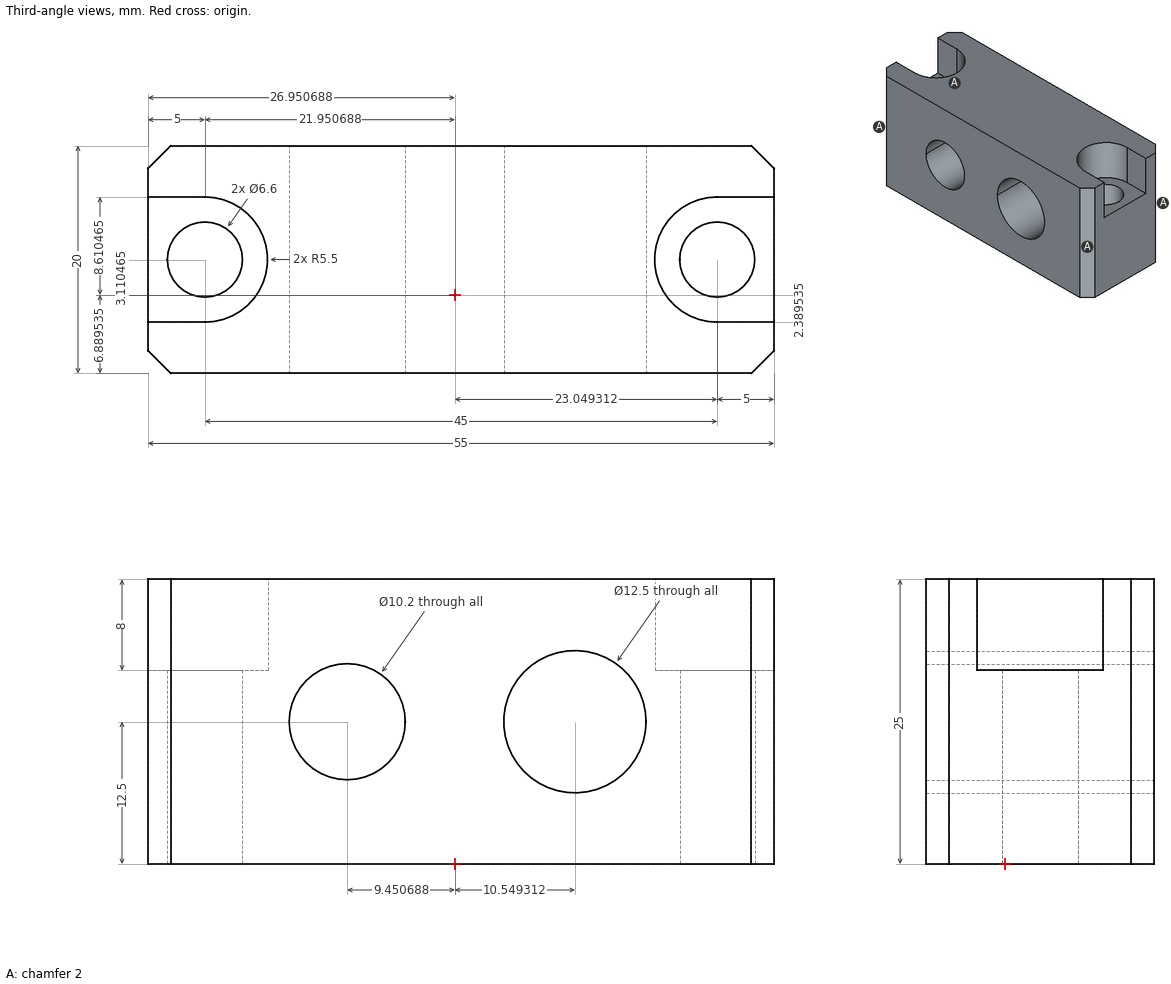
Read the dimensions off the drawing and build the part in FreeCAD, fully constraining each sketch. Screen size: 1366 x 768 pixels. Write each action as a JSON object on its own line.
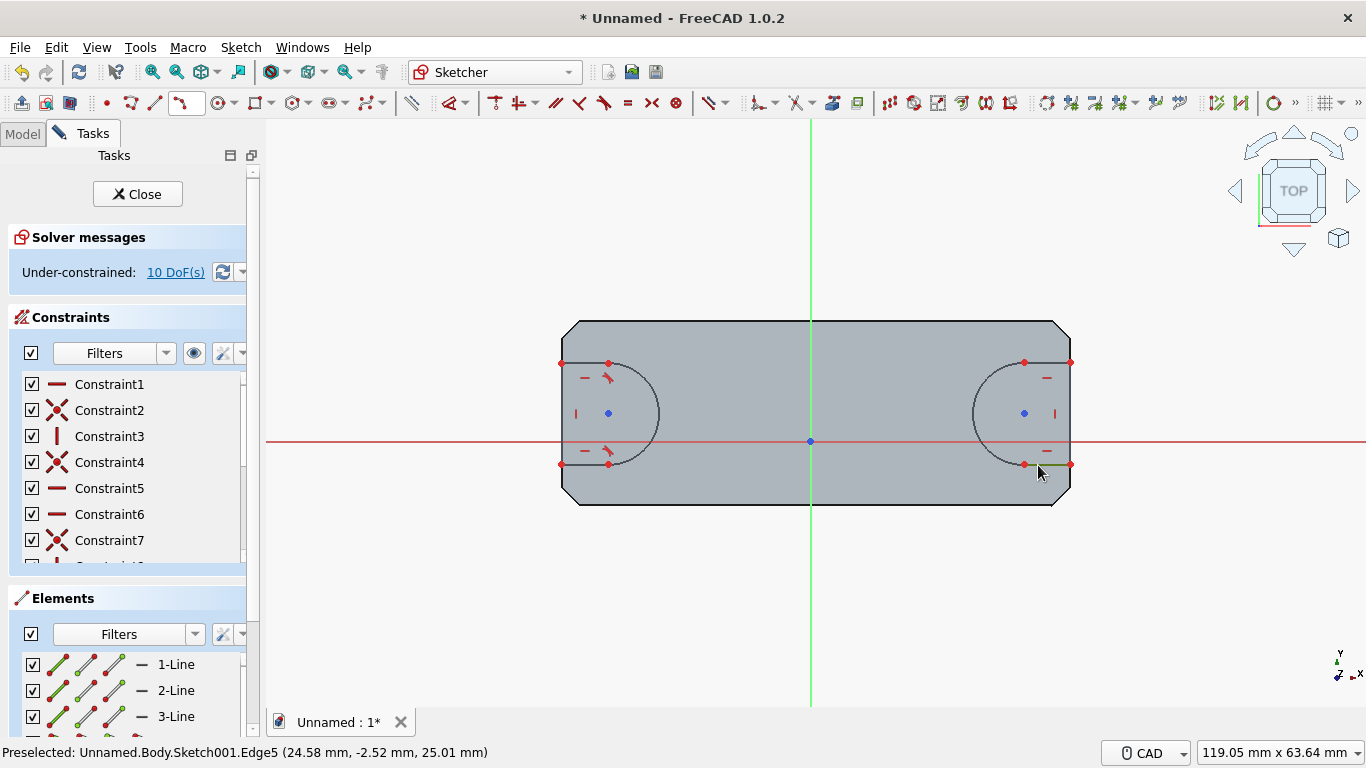
{"action": "left_click", "coordinate": [983, 384]}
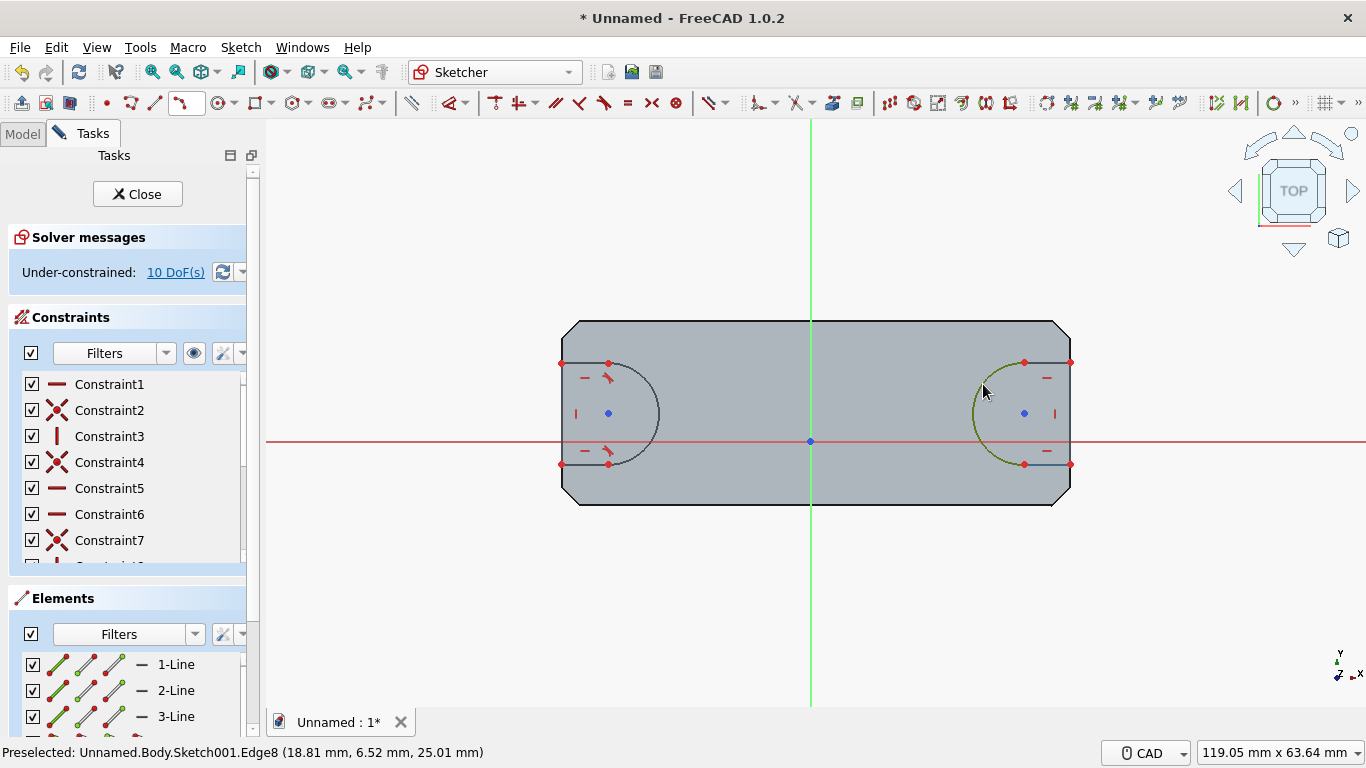
{"action": "left_click", "coordinate": [604, 104]}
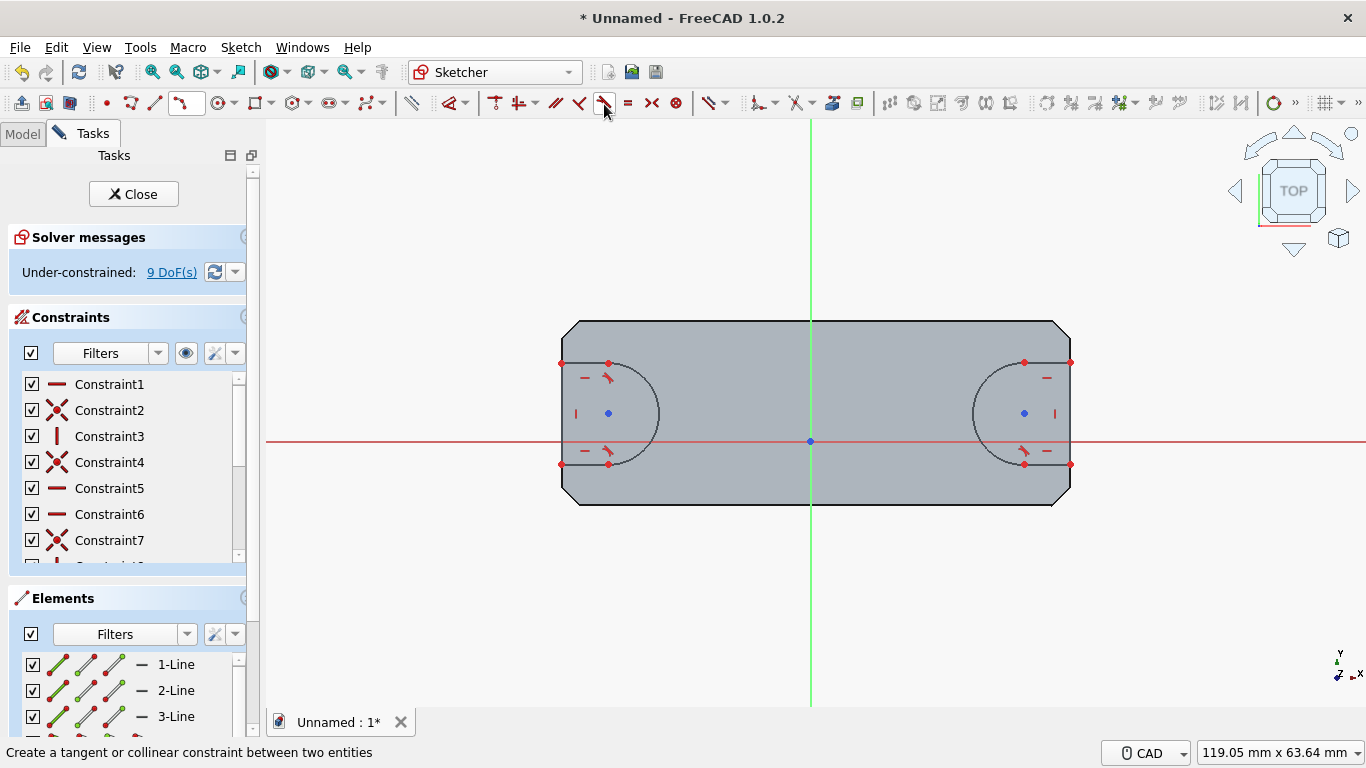
{"action": "left_click", "coordinate": [1056, 363]}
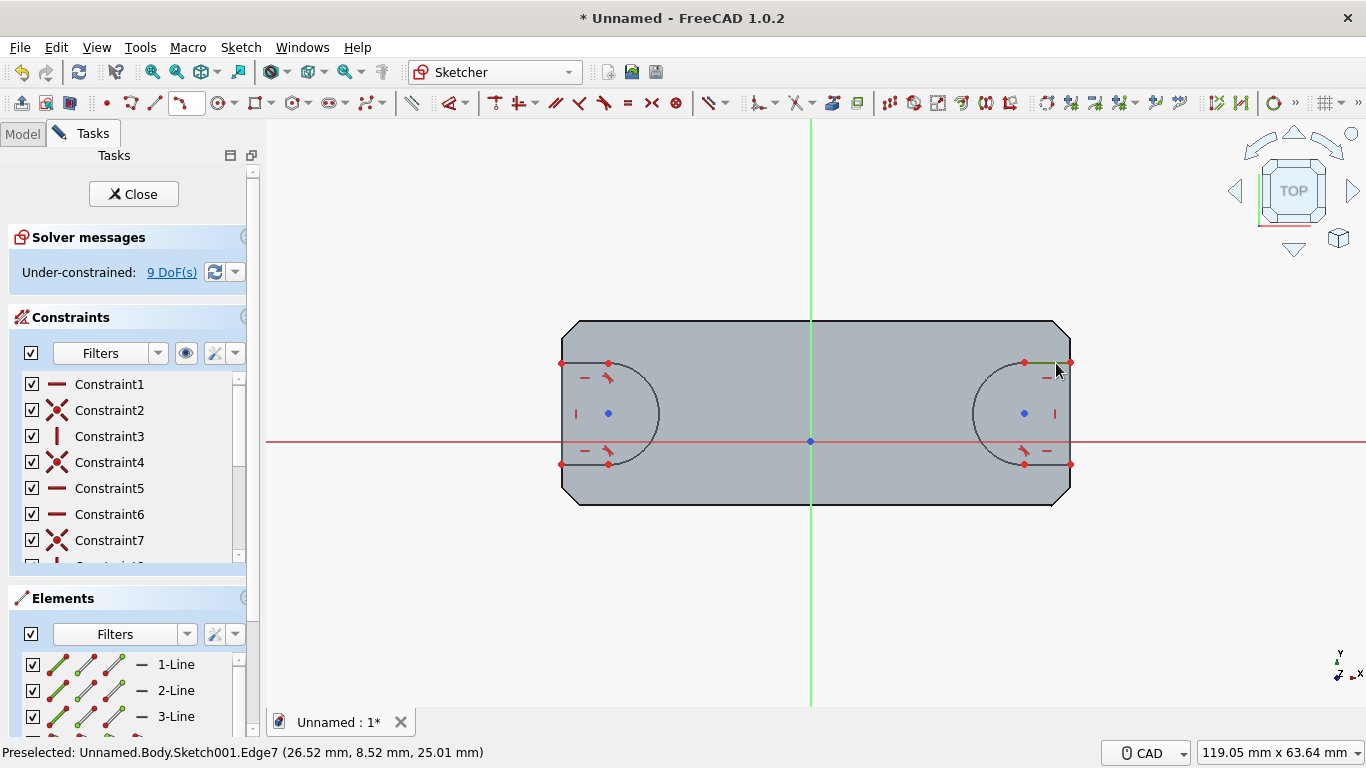
{"action": "left_click", "coordinate": [983, 384]}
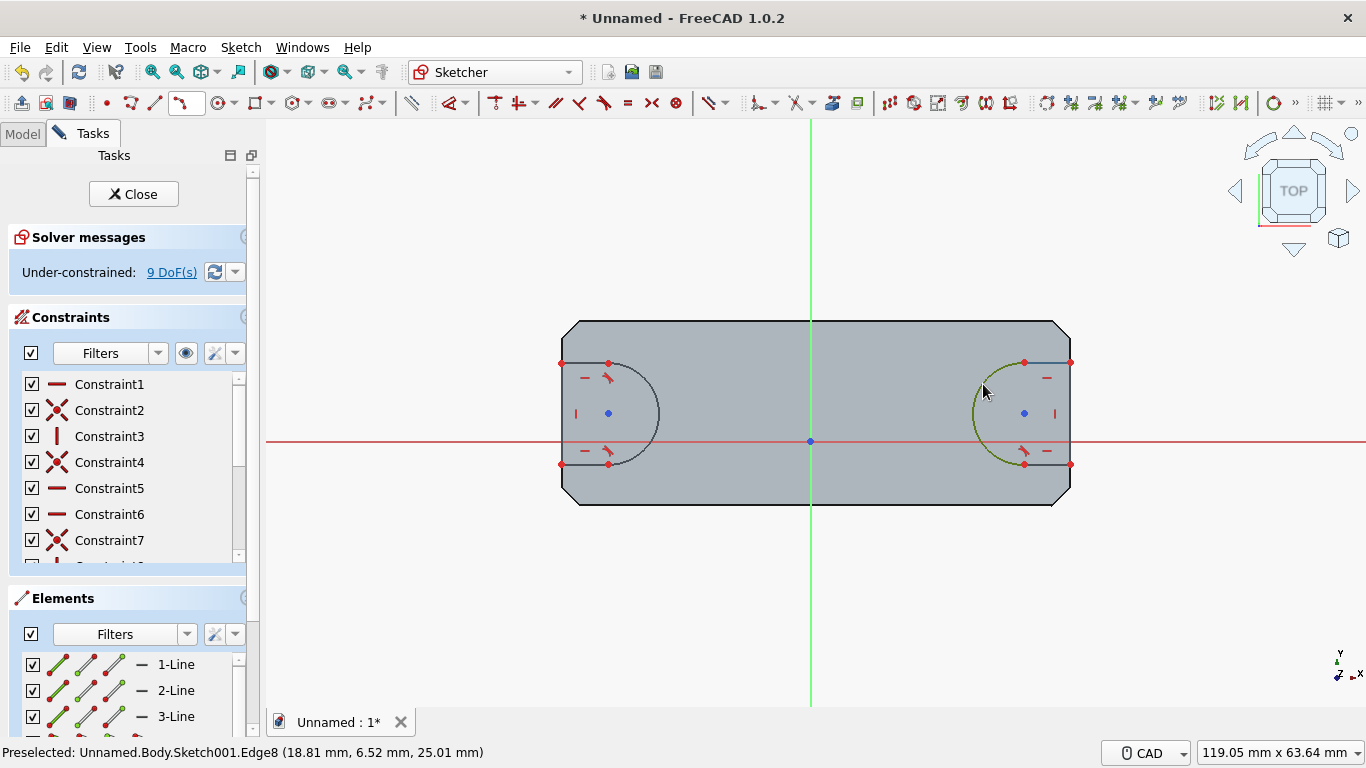
{"action": "key", "text": "t"}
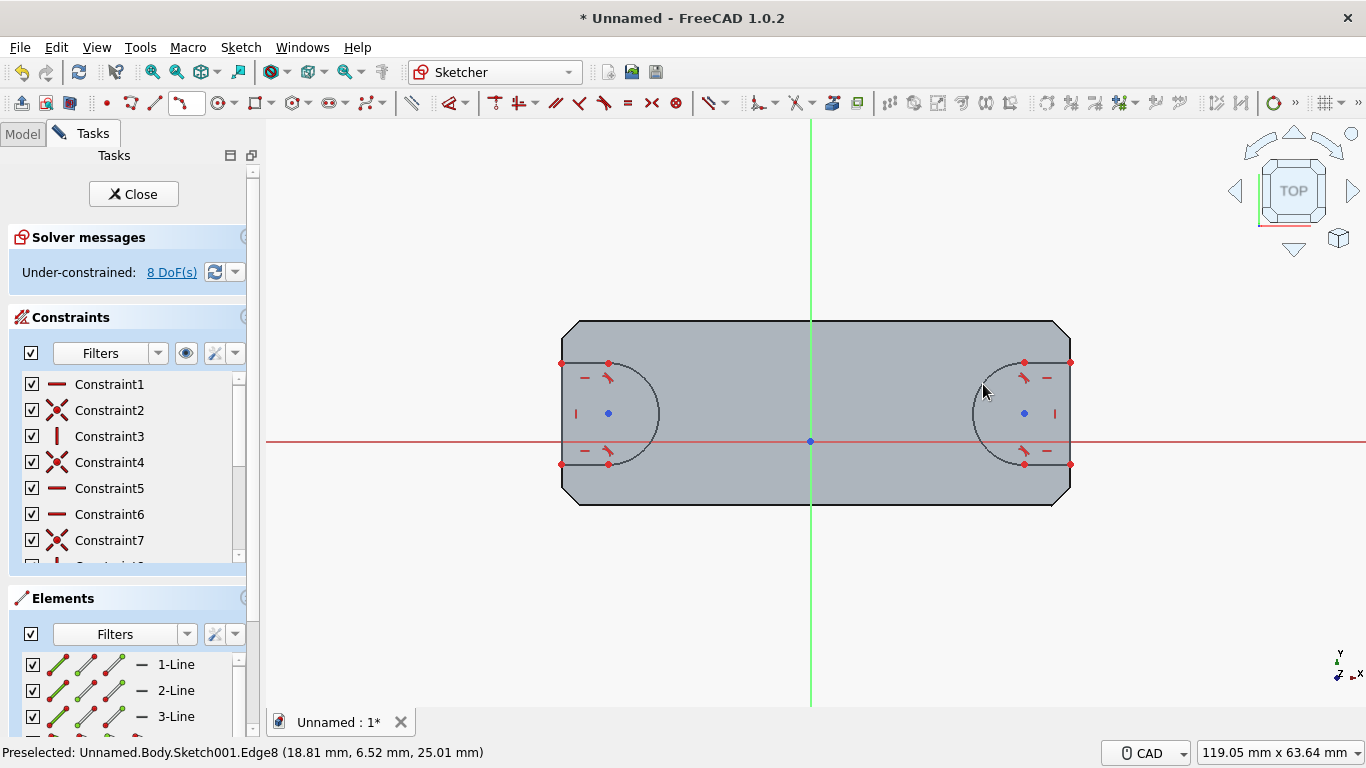
{"action": "left_click", "coordinate": [649, 444]}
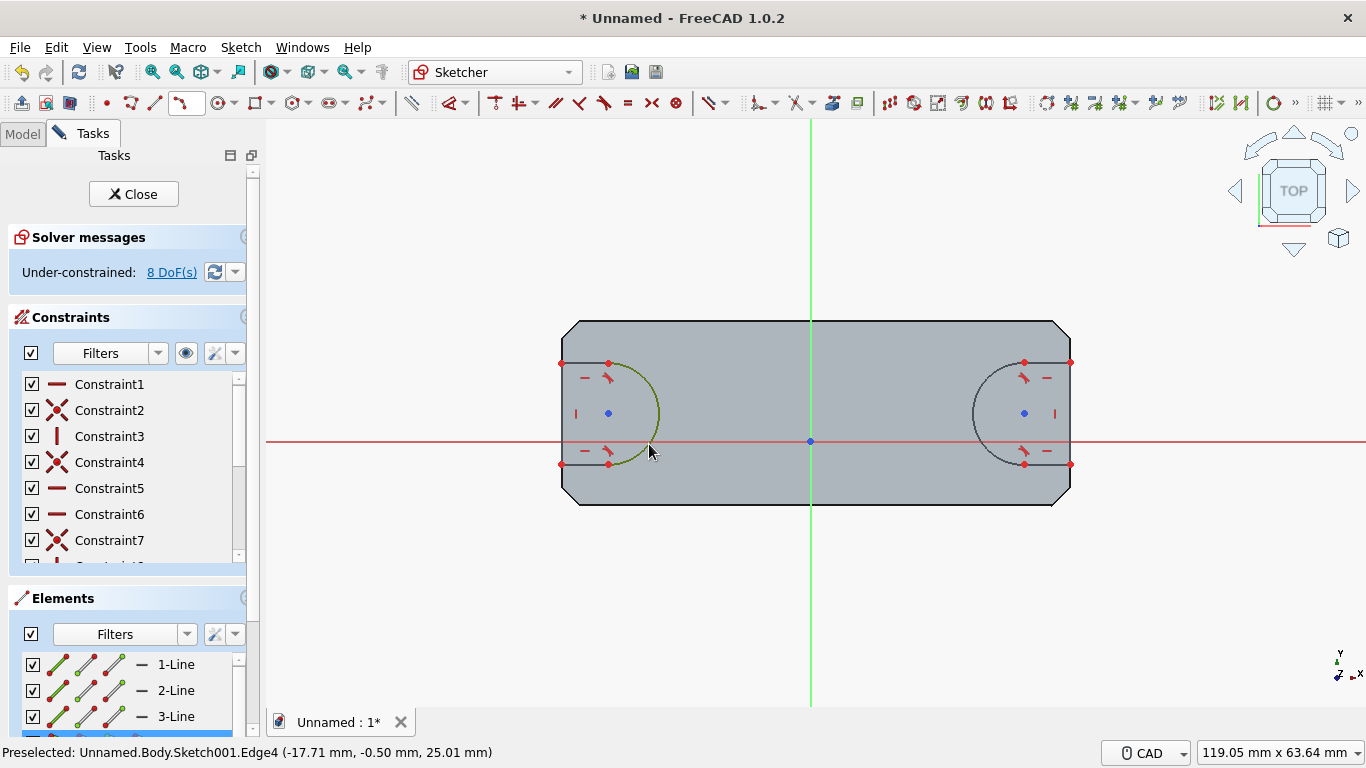
{"action": "left_click", "coordinate": [983, 384]}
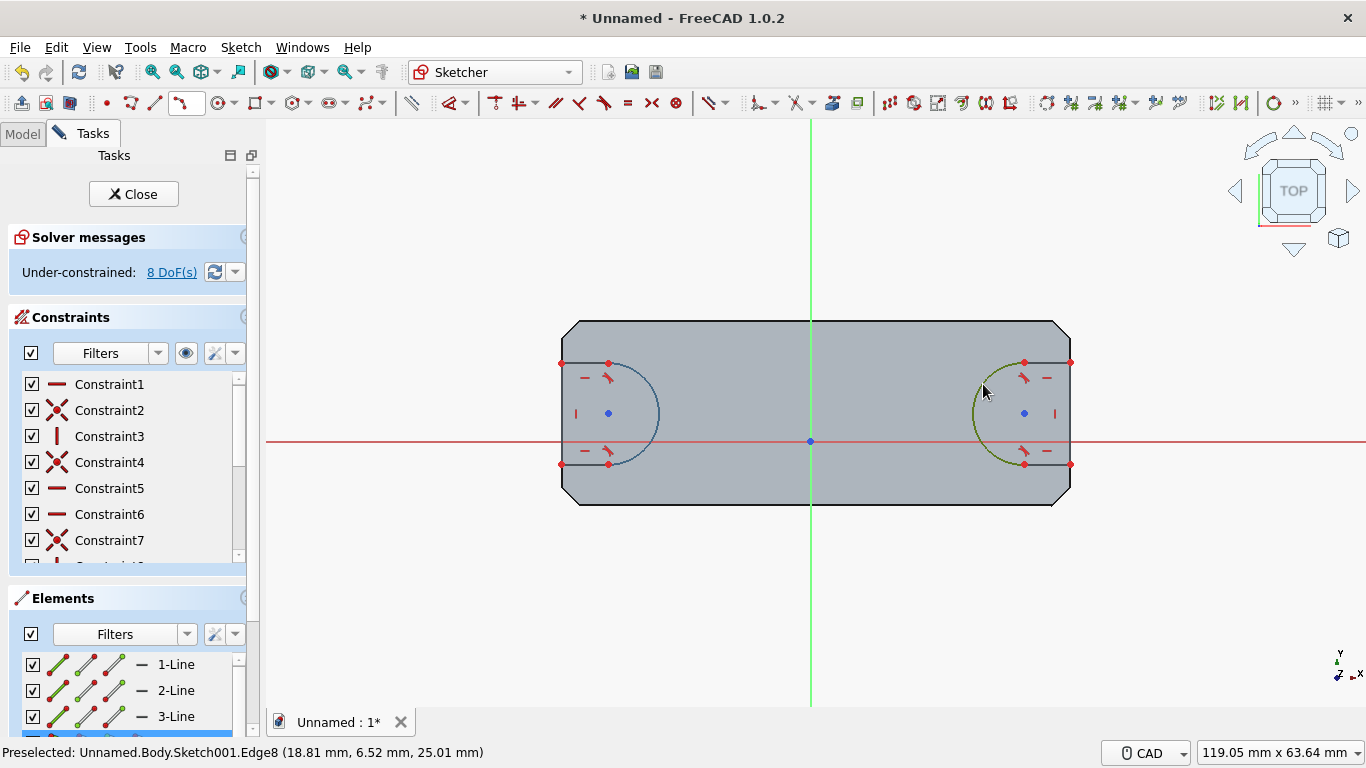
{"action": "left_click", "coordinate": [628, 104]}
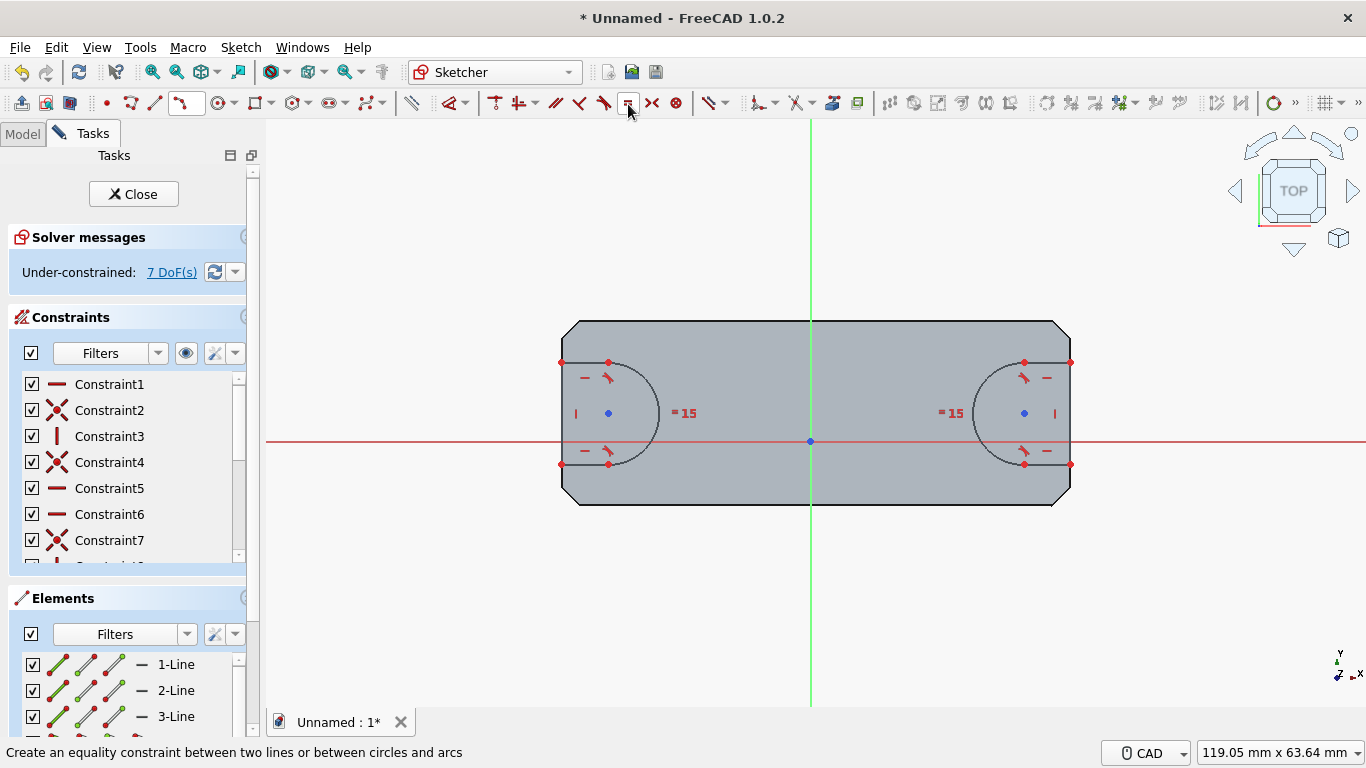
{"action": "left_click", "coordinate": [450, 104]}